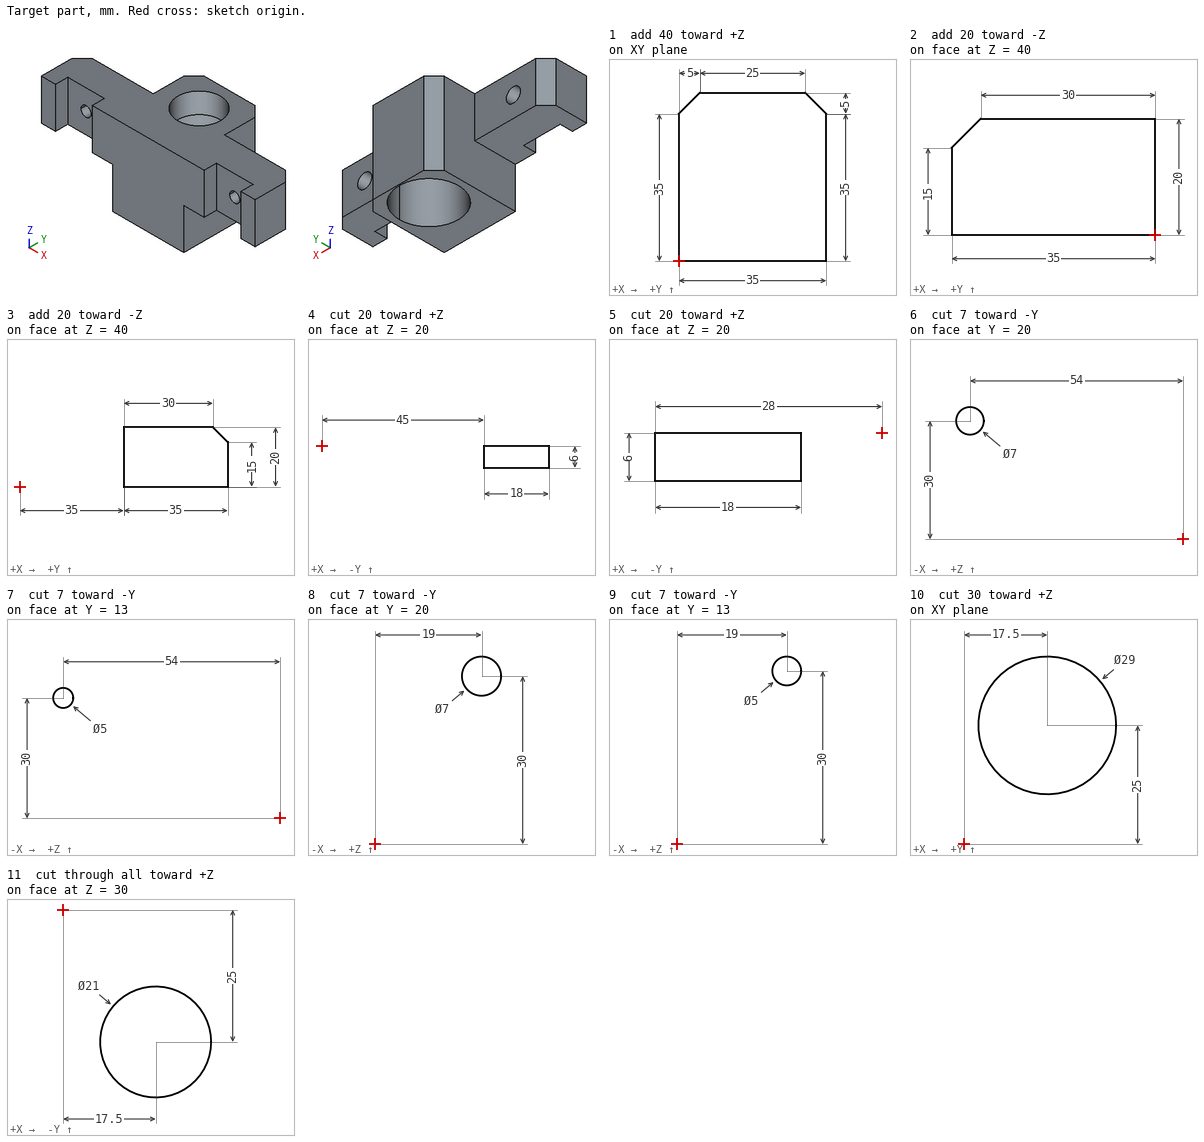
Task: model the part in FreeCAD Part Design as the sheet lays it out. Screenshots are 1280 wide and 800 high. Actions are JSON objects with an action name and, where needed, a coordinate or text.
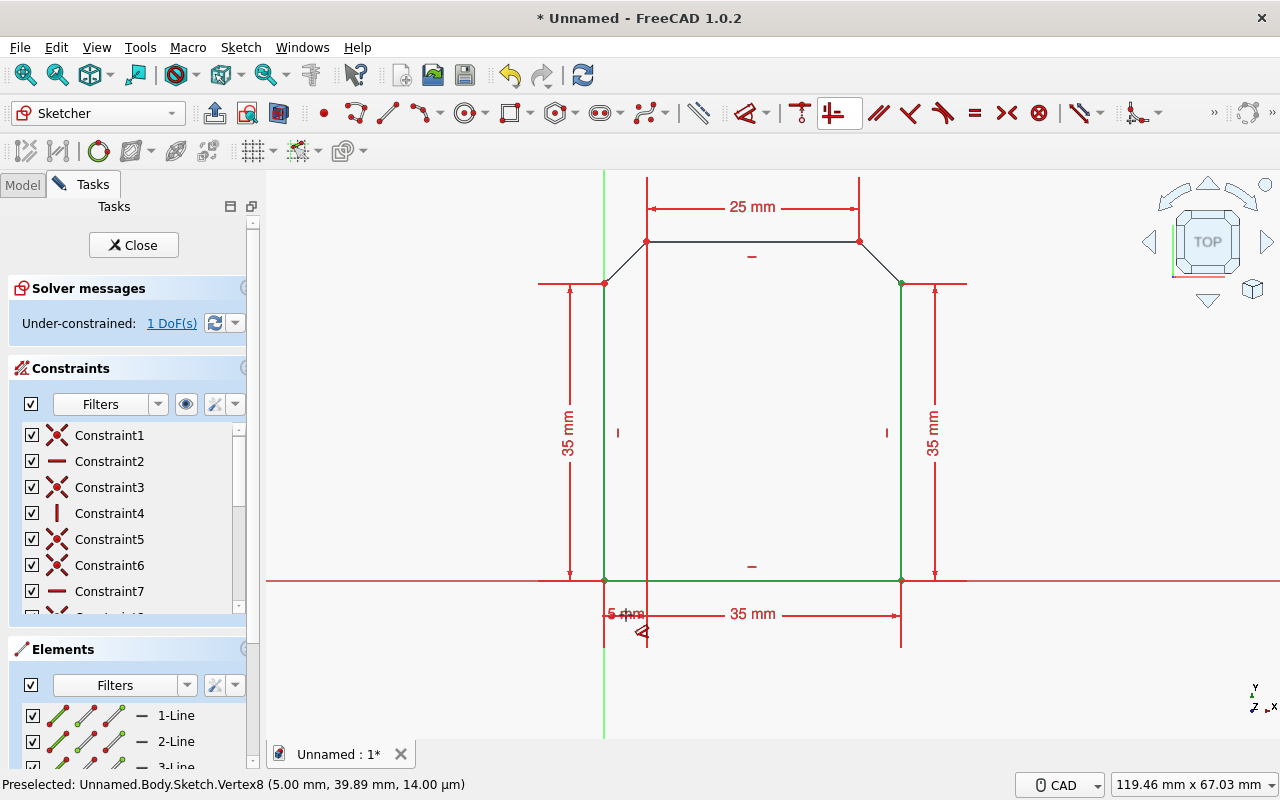
{"action": "left_click", "coordinate": [889, 271]}
{"action": "left_click", "coordinate": [935, 263]}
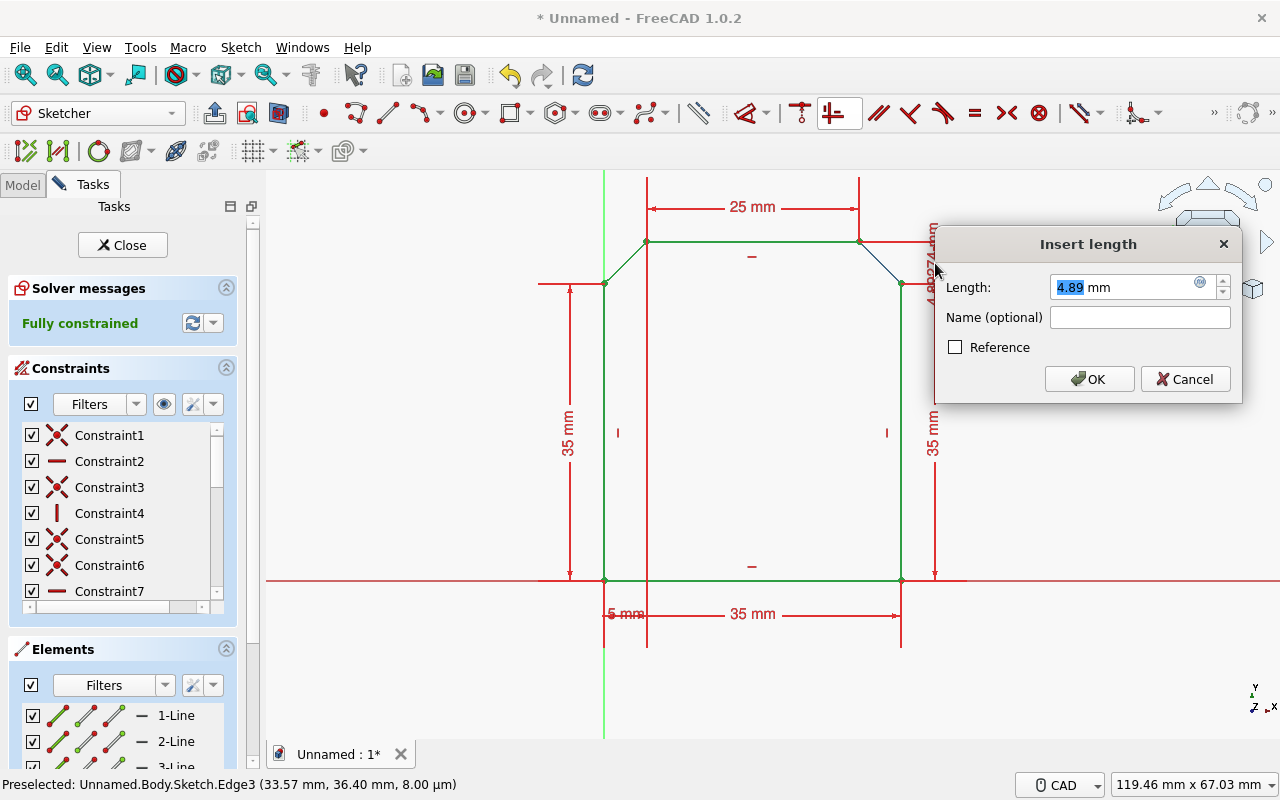
{"action": "type", "text": "5"}
{"action": "key", "text": "Return"}
{"action": "key", "text": "Escape"}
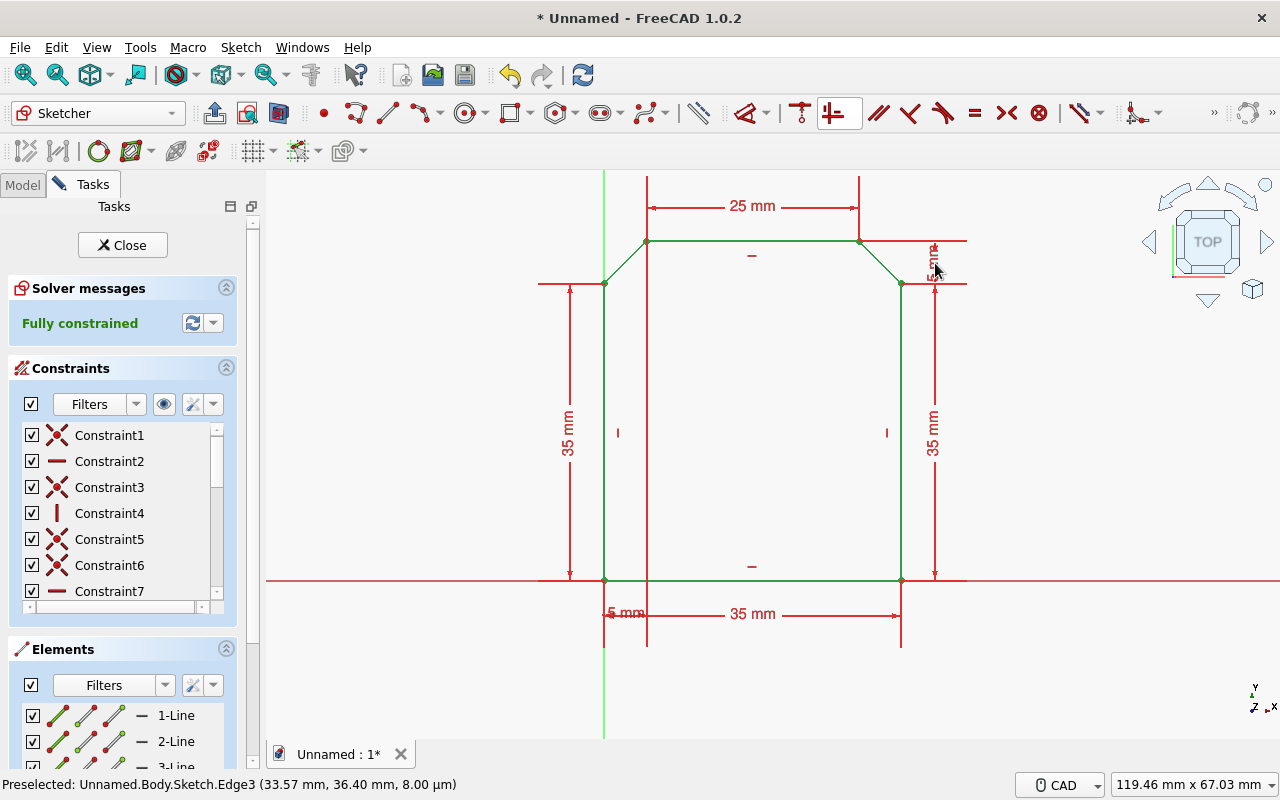
{"action": "left_click", "coordinate": [123, 245]}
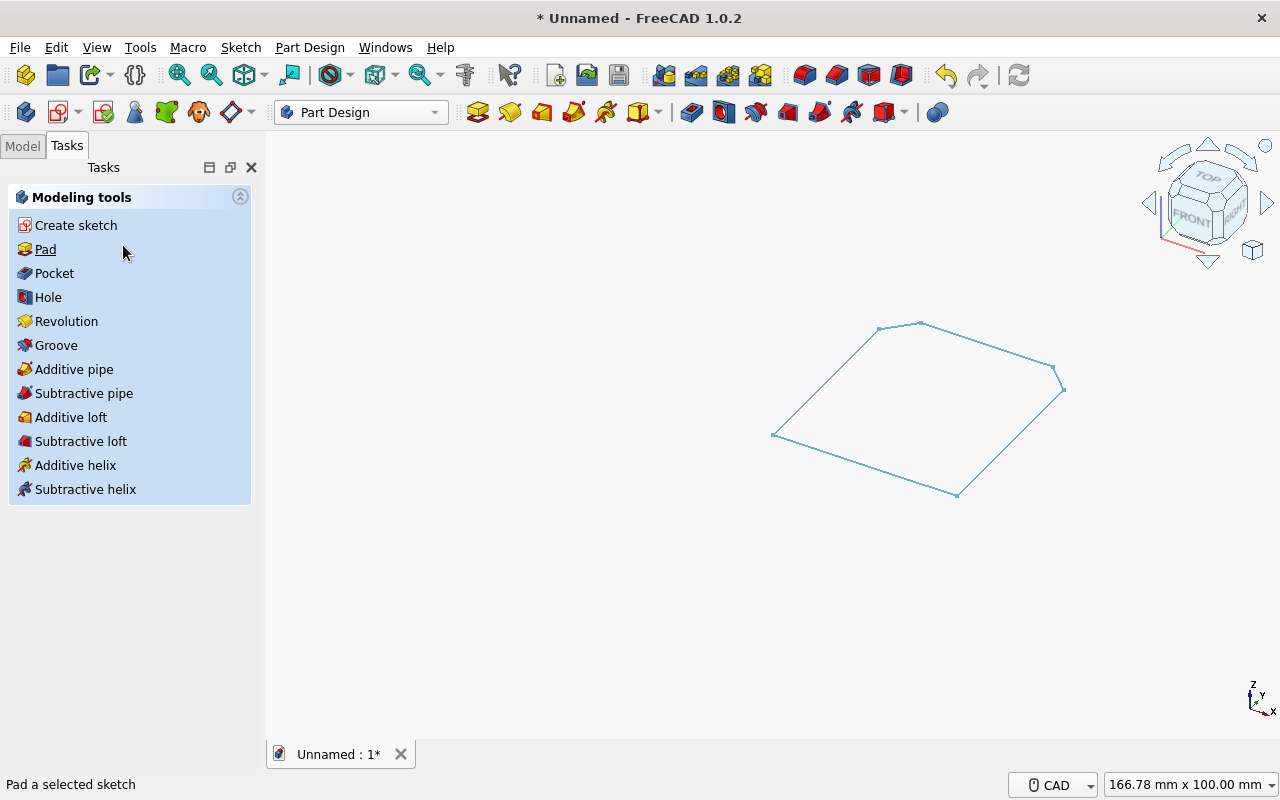
{"action": "left_click", "coordinate": [478, 112]}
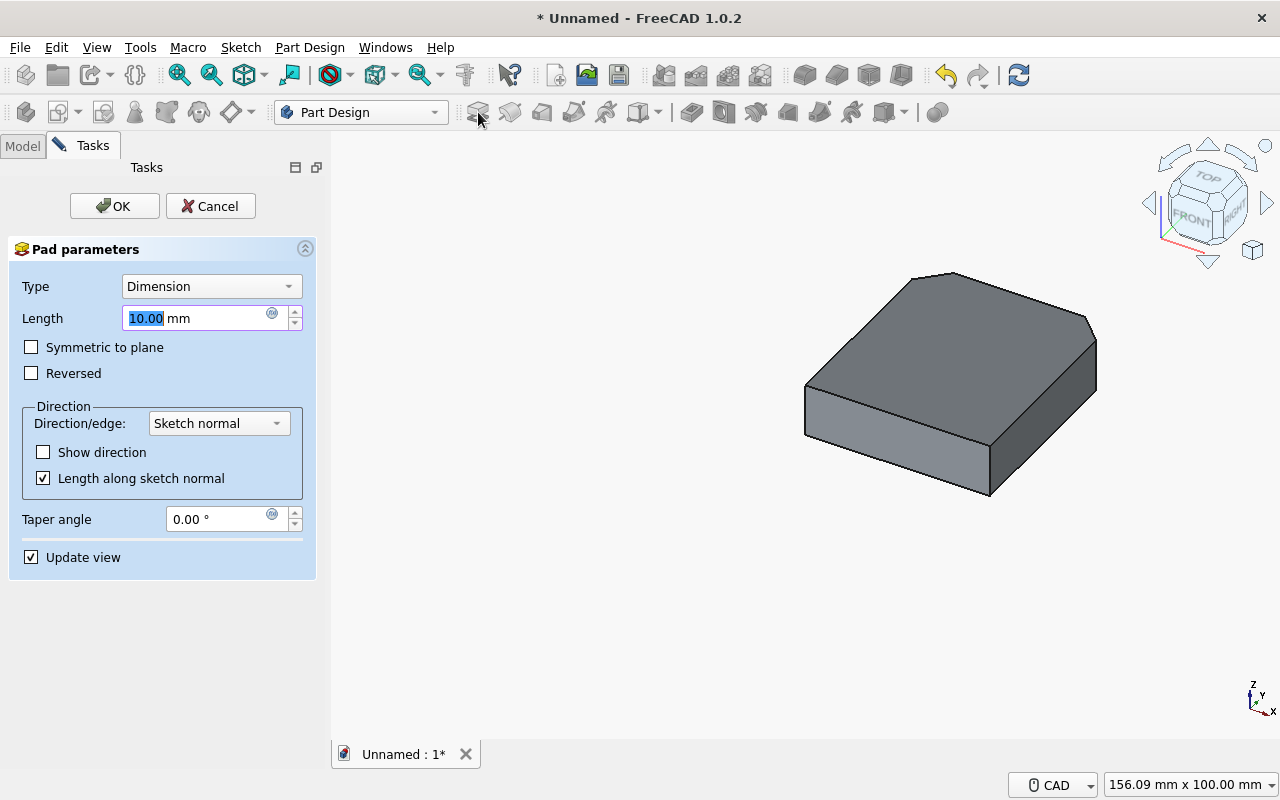
{"action": "type", "text": "40"}
{"action": "key", "text": "Tab"}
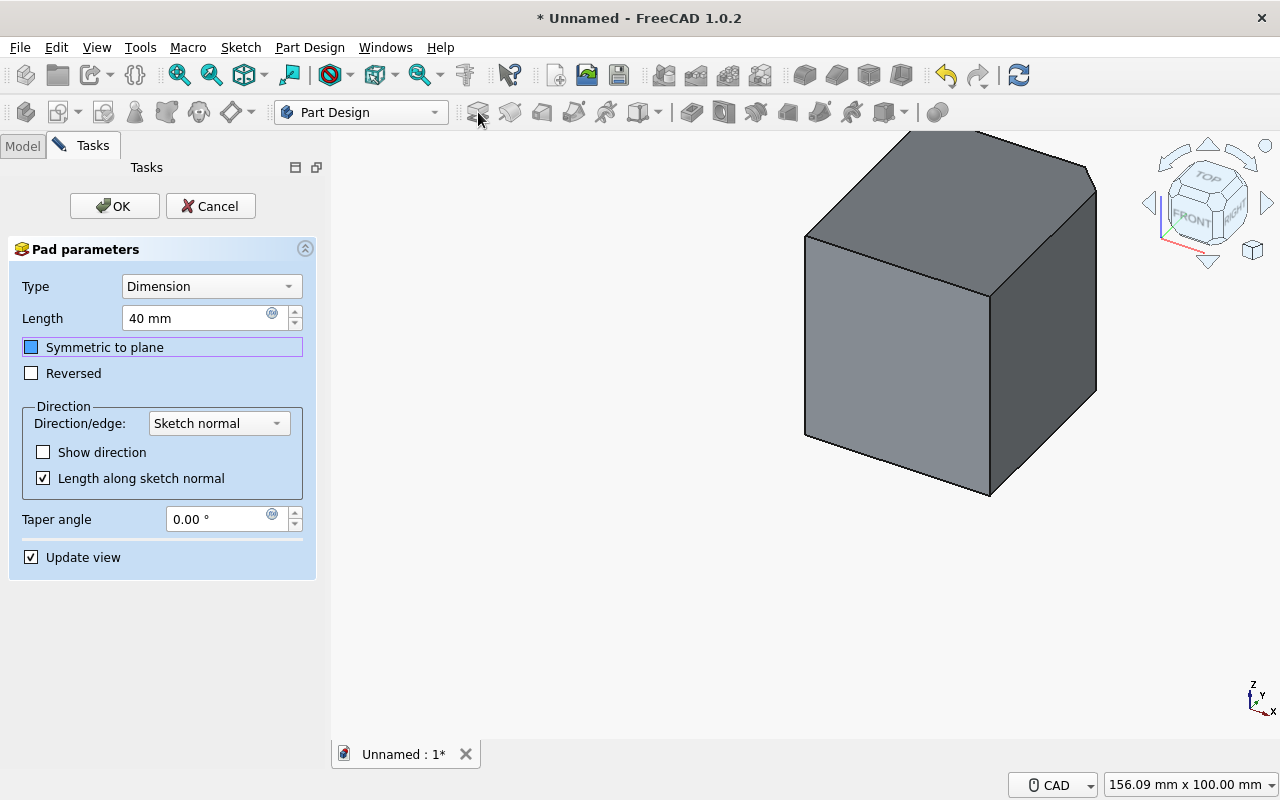
{"action": "left_click", "coordinate": [115, 206]}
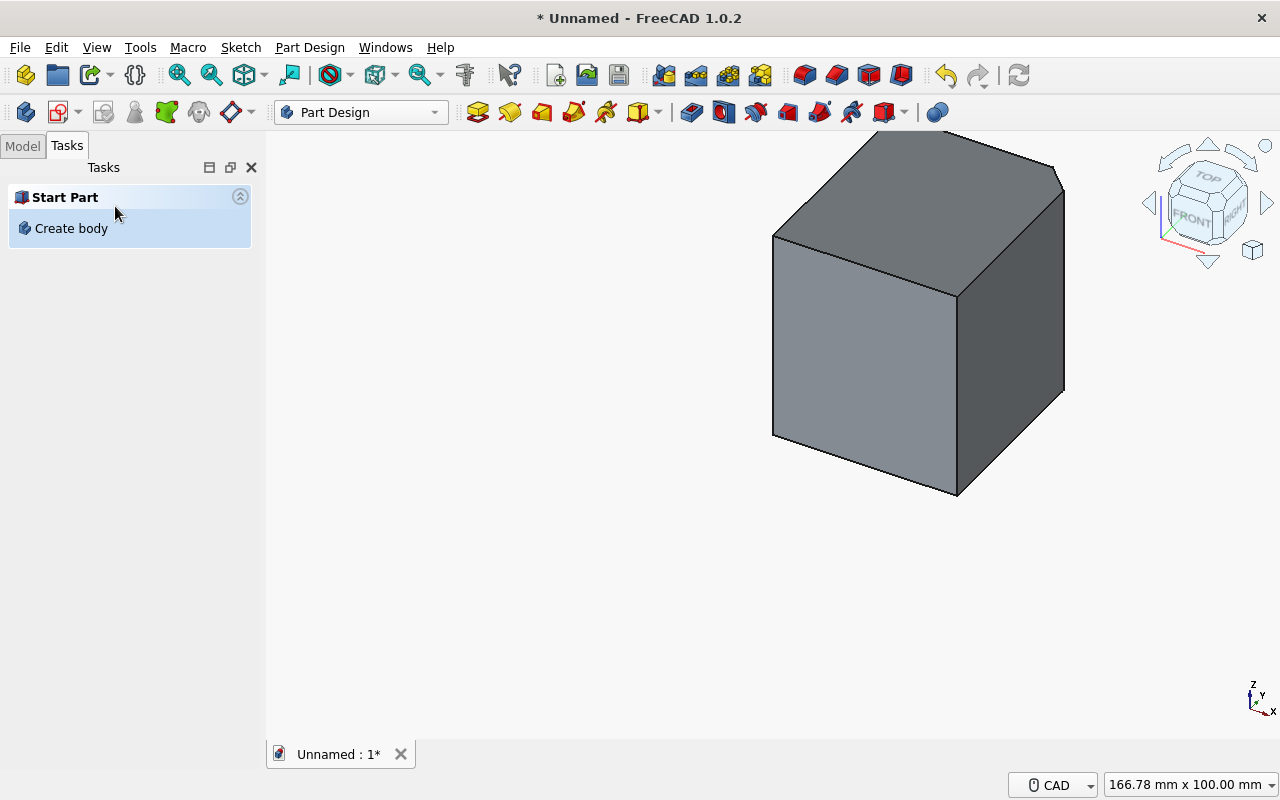
{"action": "left_click", "coordinate": [180, 76]}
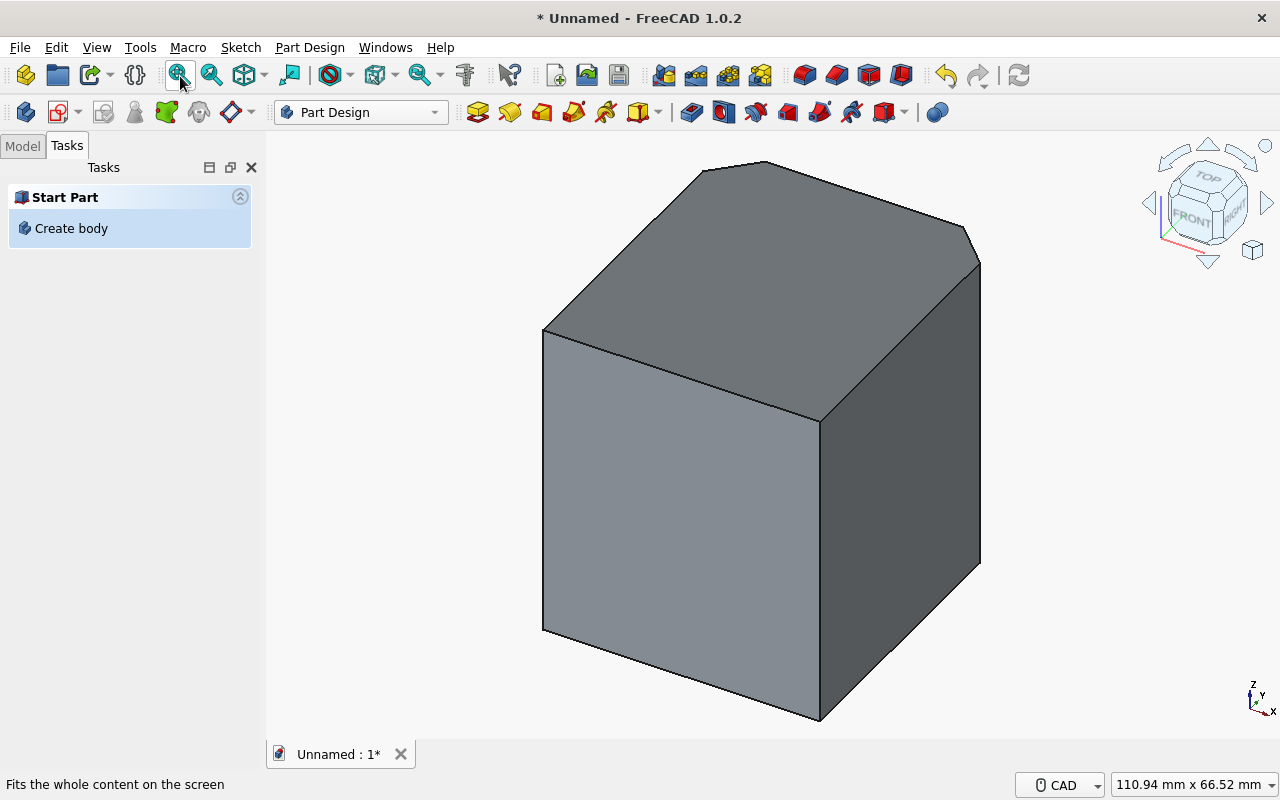
{"action": "left_click", "coordinate": [773, 284]}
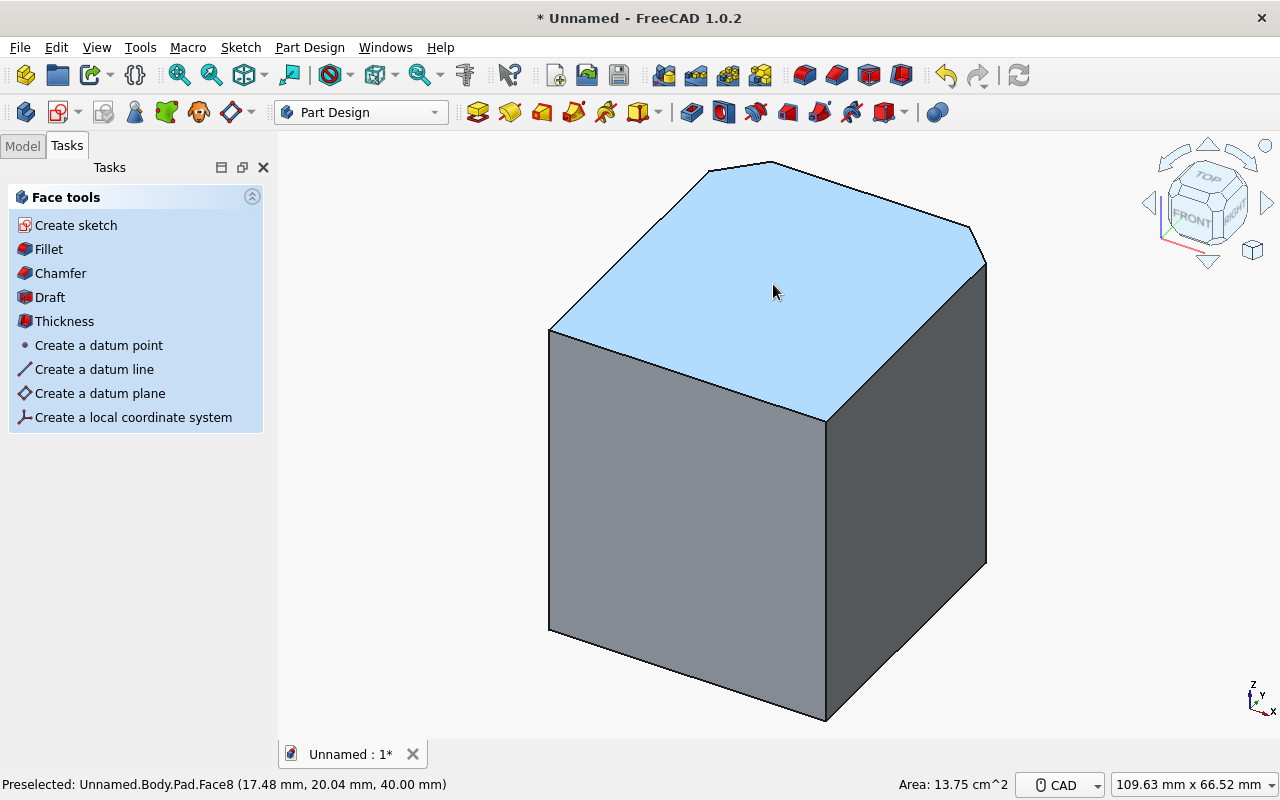
{"action": "left_click", "coordinate": [58, 112]}